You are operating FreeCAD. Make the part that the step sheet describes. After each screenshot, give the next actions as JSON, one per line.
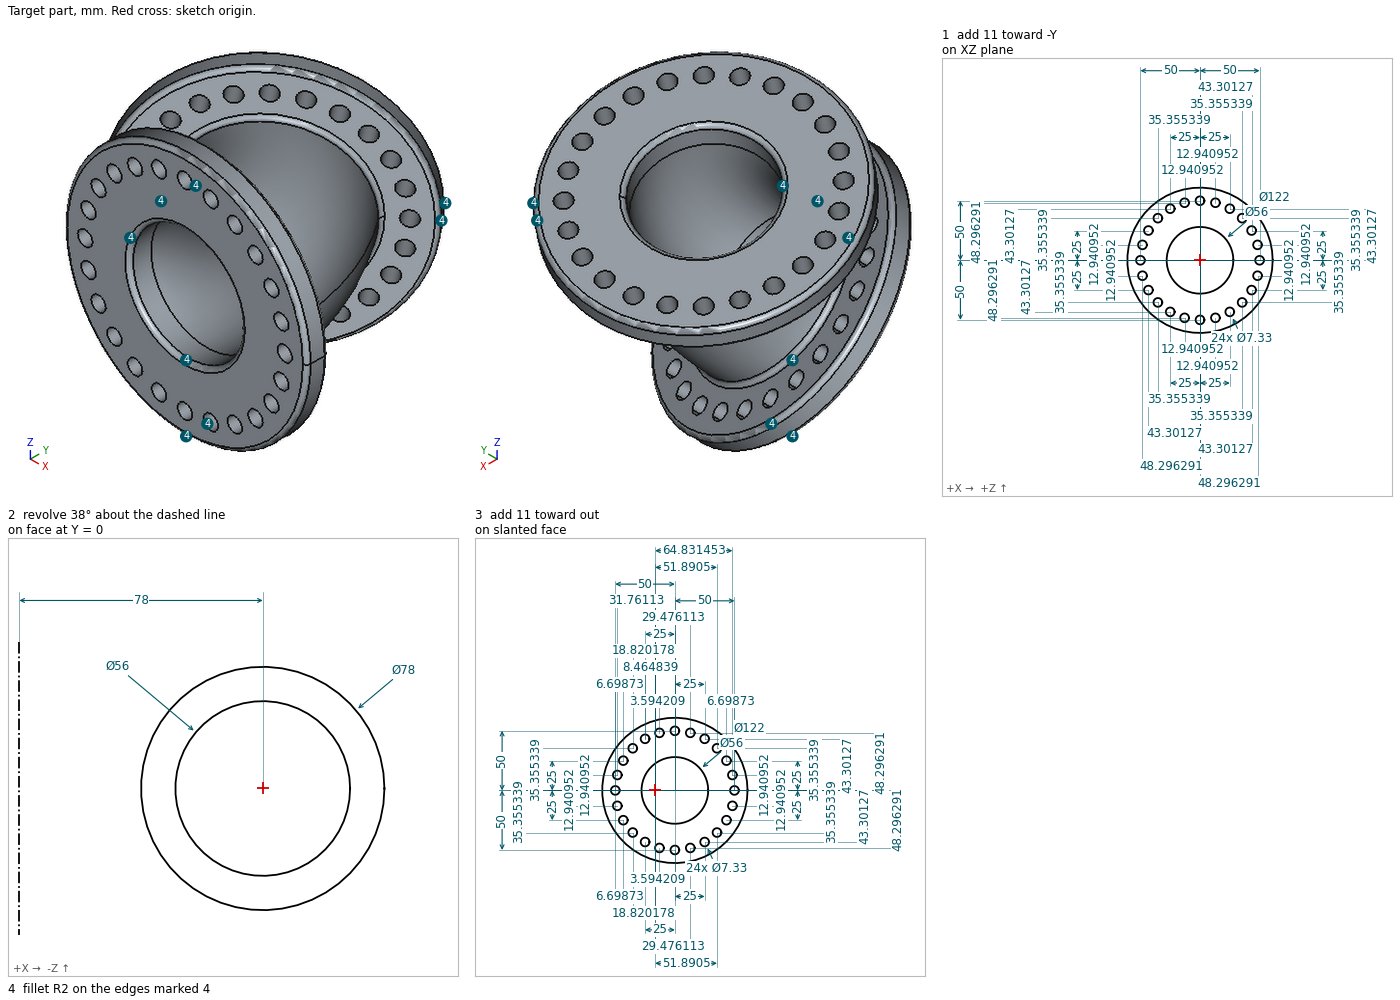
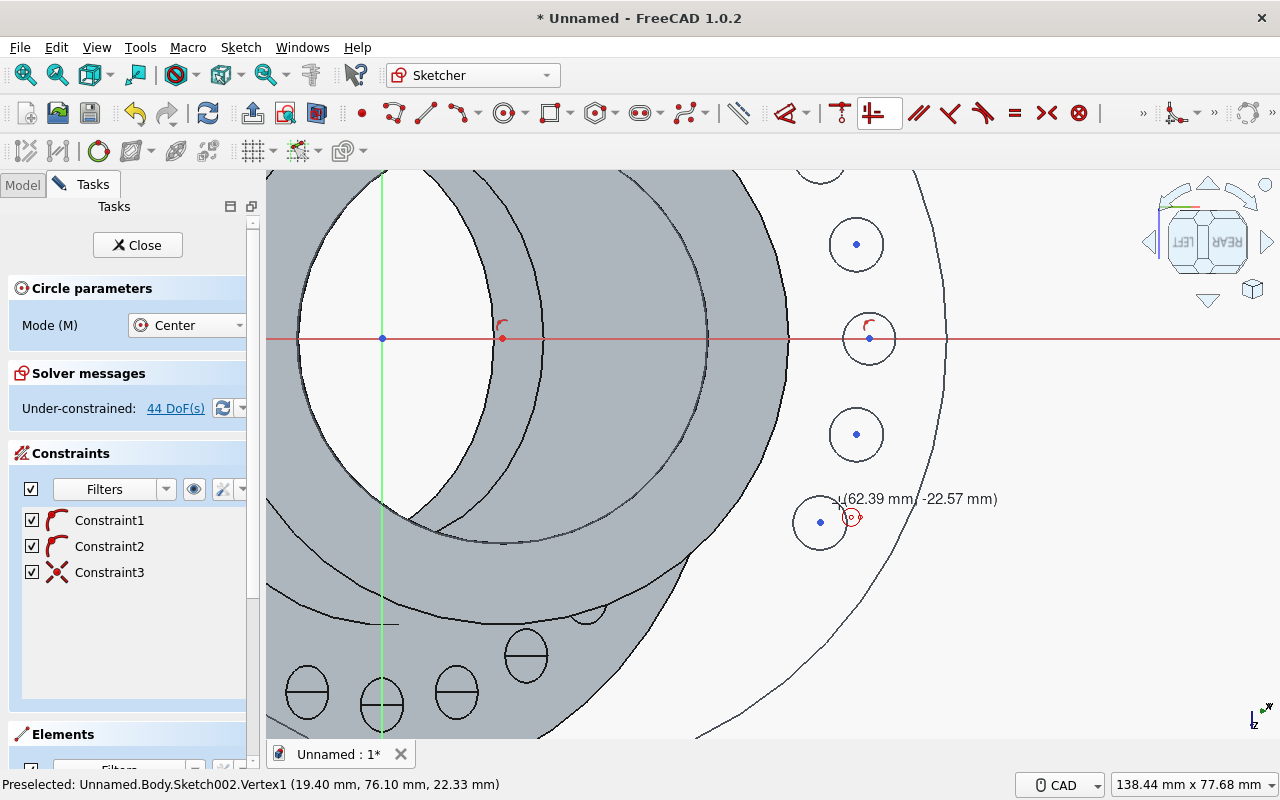
{"action": "left_click", "coordinate": [762, 598]}
{"action": "left_click", "coordinate": [781, 579]}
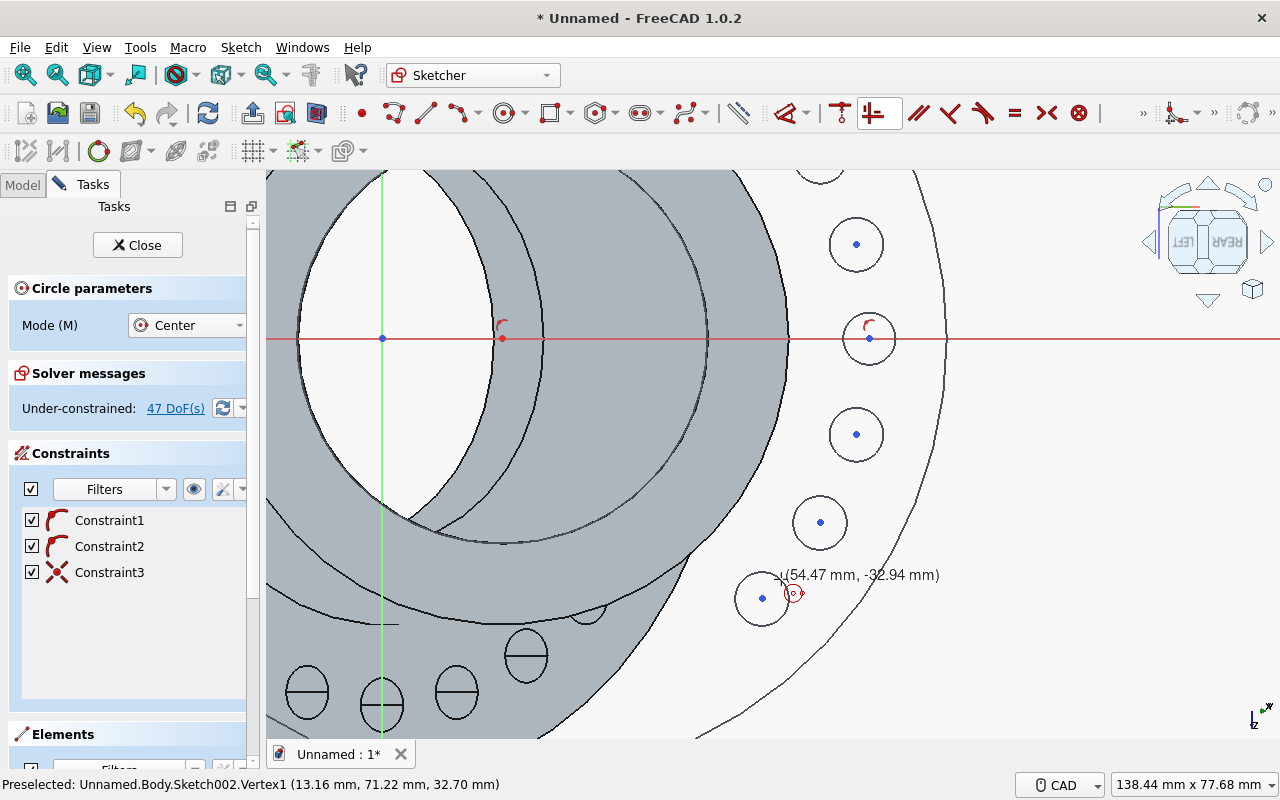
{"action": "left_click", "coordinate": [686, 656]}
{"action": "left_click", "coordinate": [705, 637]}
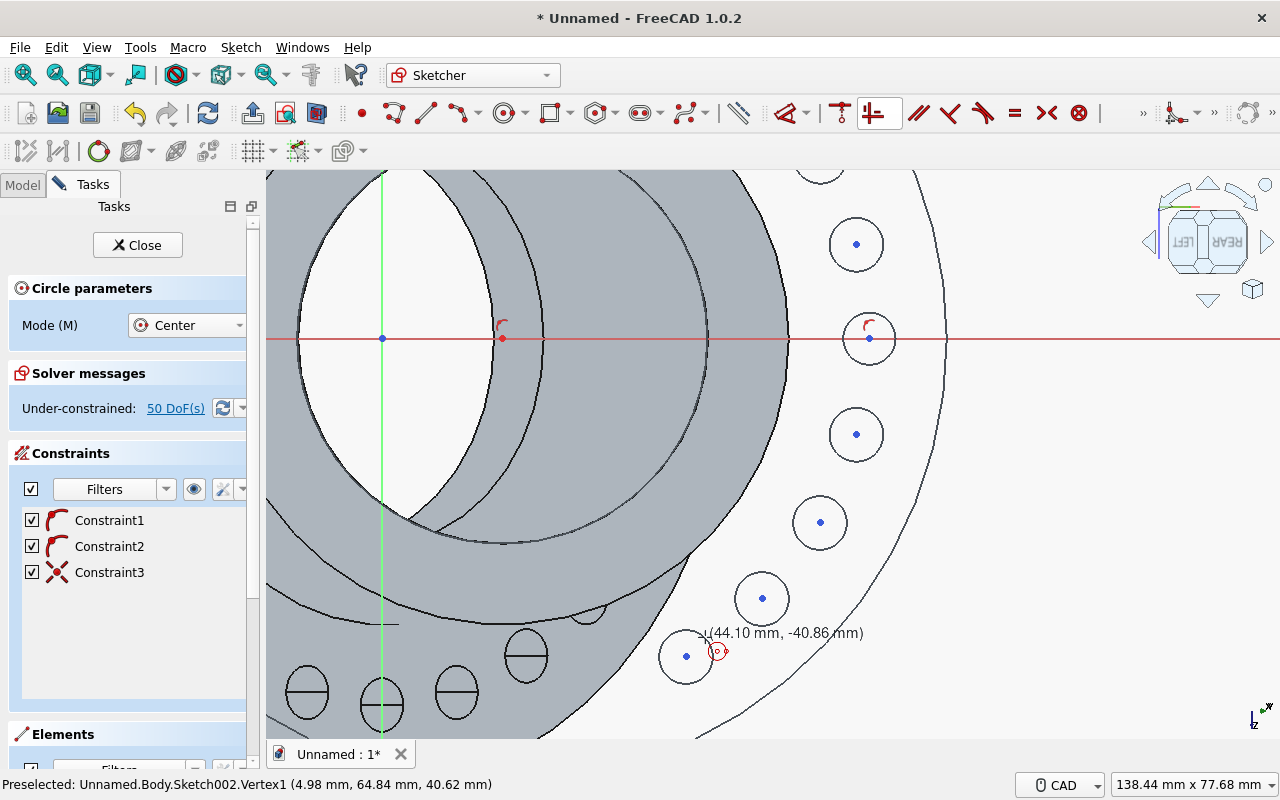
{"action": "left_click", "coordinate": [598, 692]}
{"action": "left_click", "coordinate": [617, 673]}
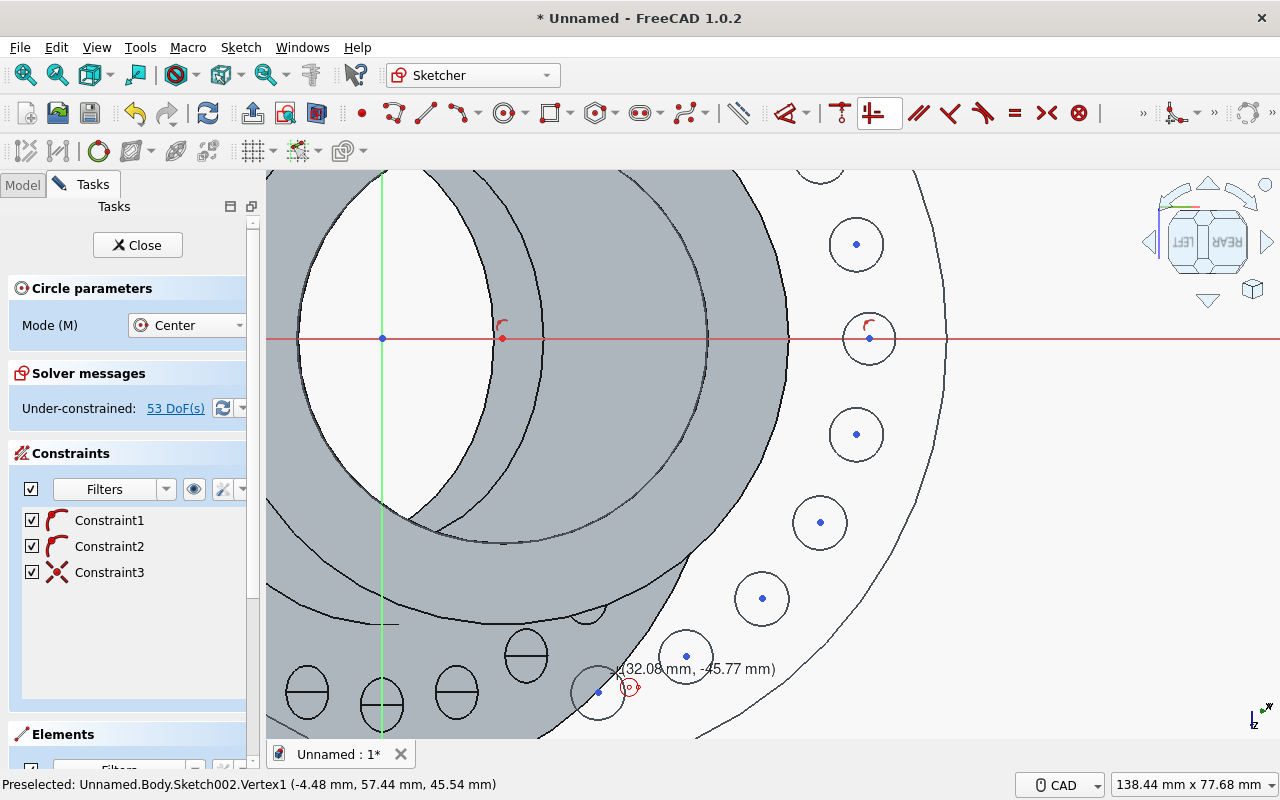
{"action": "left_click", "coordinate": [503, 705]}
{"action": "left_click", "coordinate": [522, 686]}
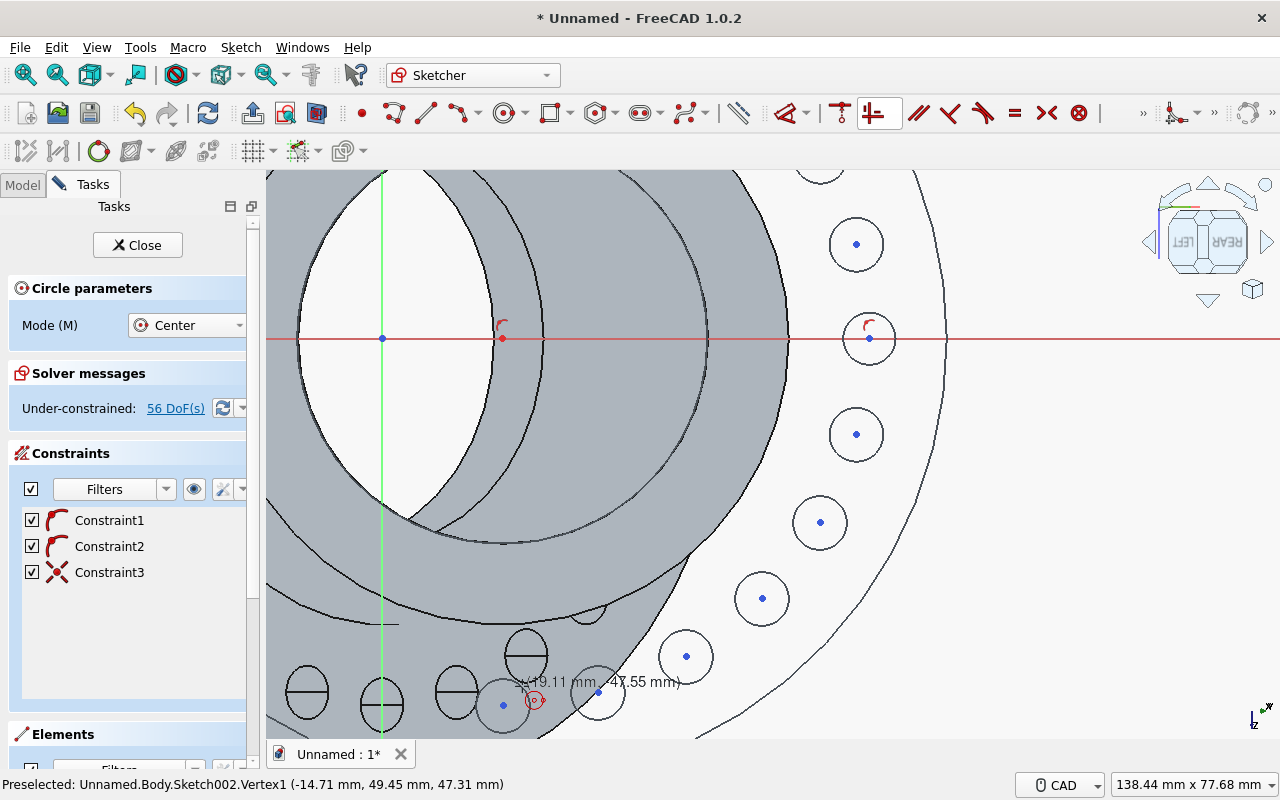
{"action": "scroll", "coordinate": [822, 522], "scroll_direction": "down", "scroll_amount": 5}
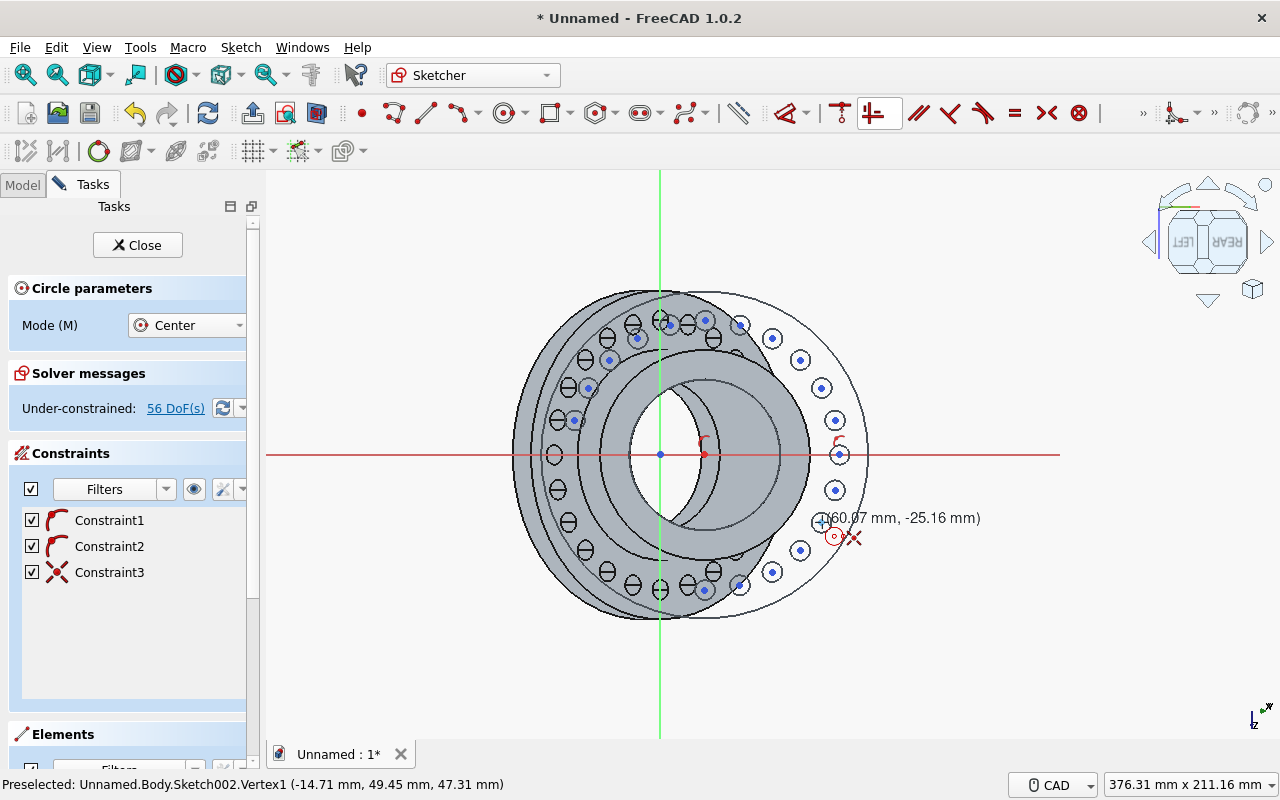
{"action": "scroll", "coordinate": [570, 455], "scroll_direction": "up", "scroll_amount": 5}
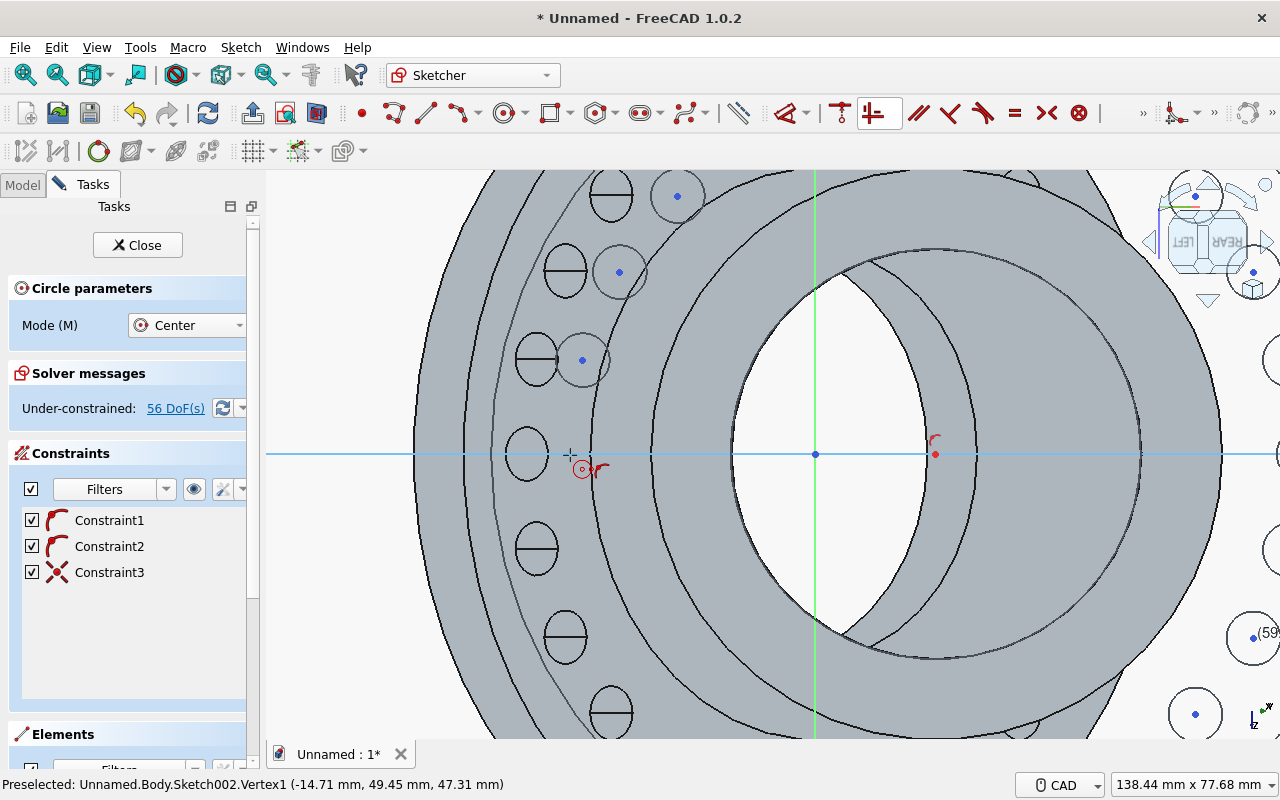
{"action": "left_click", "coordinate": [570, 454]}
{"action": "left_click", "coordinate": [589, 435]}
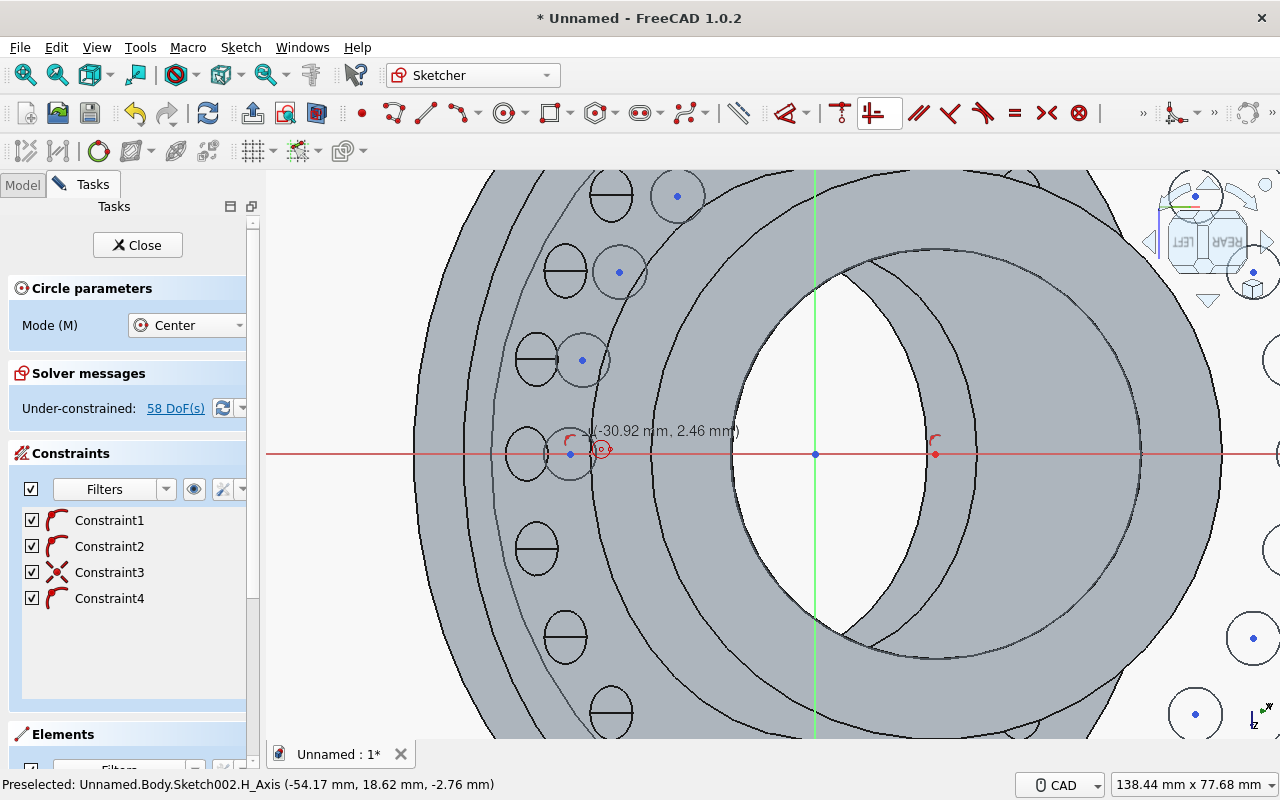
{"action": "left_click", "coordinate": [583, 549]}
{"action": "left_click", "coordinate": [602, 530]}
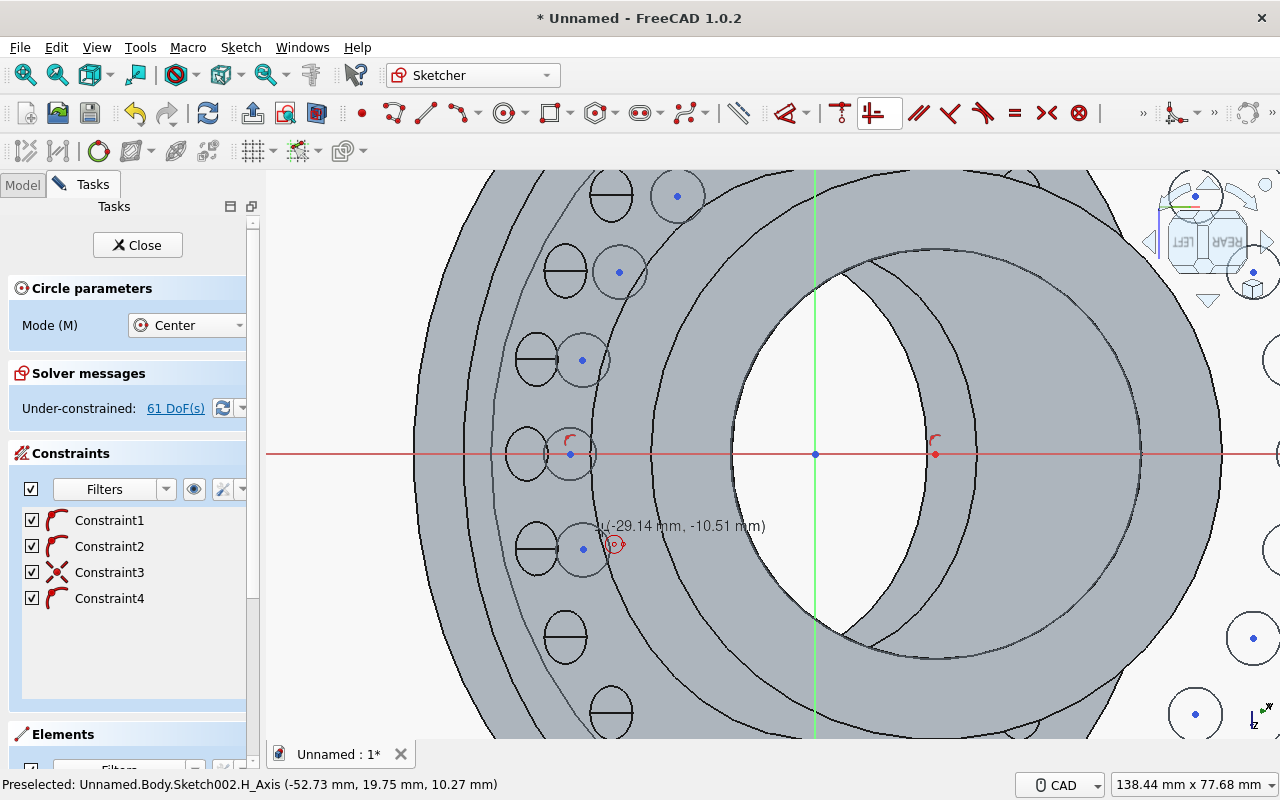
{"action": "left_click", "coordinate": [619, 637]}
{"action": "left_click", "coordinate": [638, 618]}